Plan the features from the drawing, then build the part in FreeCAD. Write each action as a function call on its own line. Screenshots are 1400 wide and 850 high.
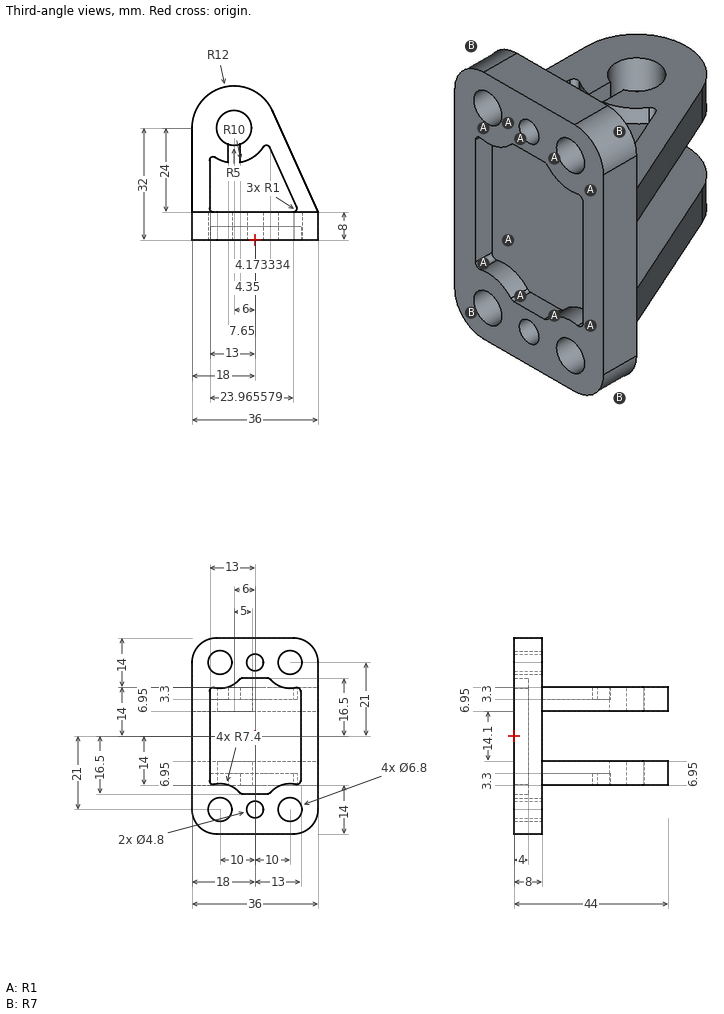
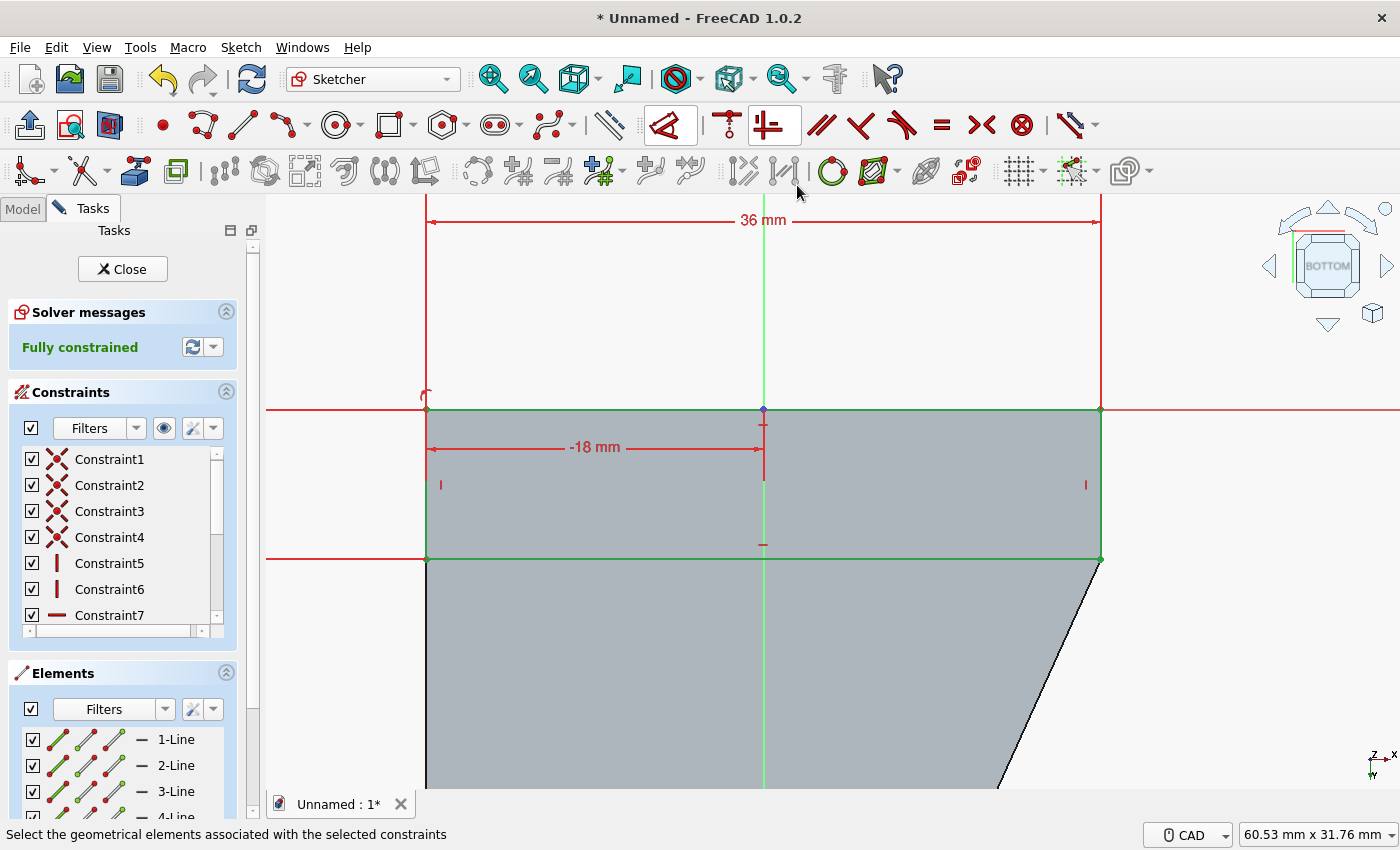
click(123, 269)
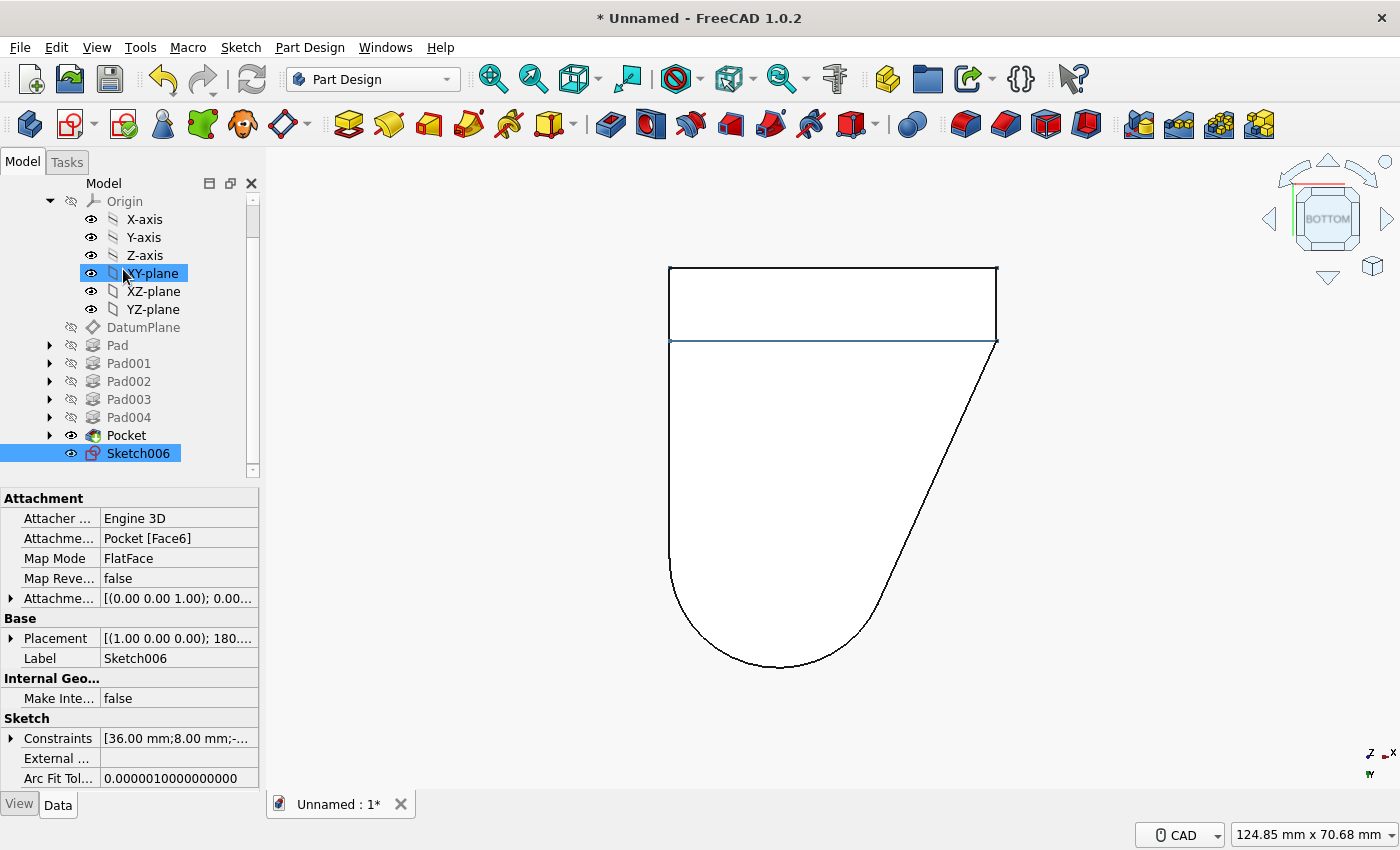
click(350, 124)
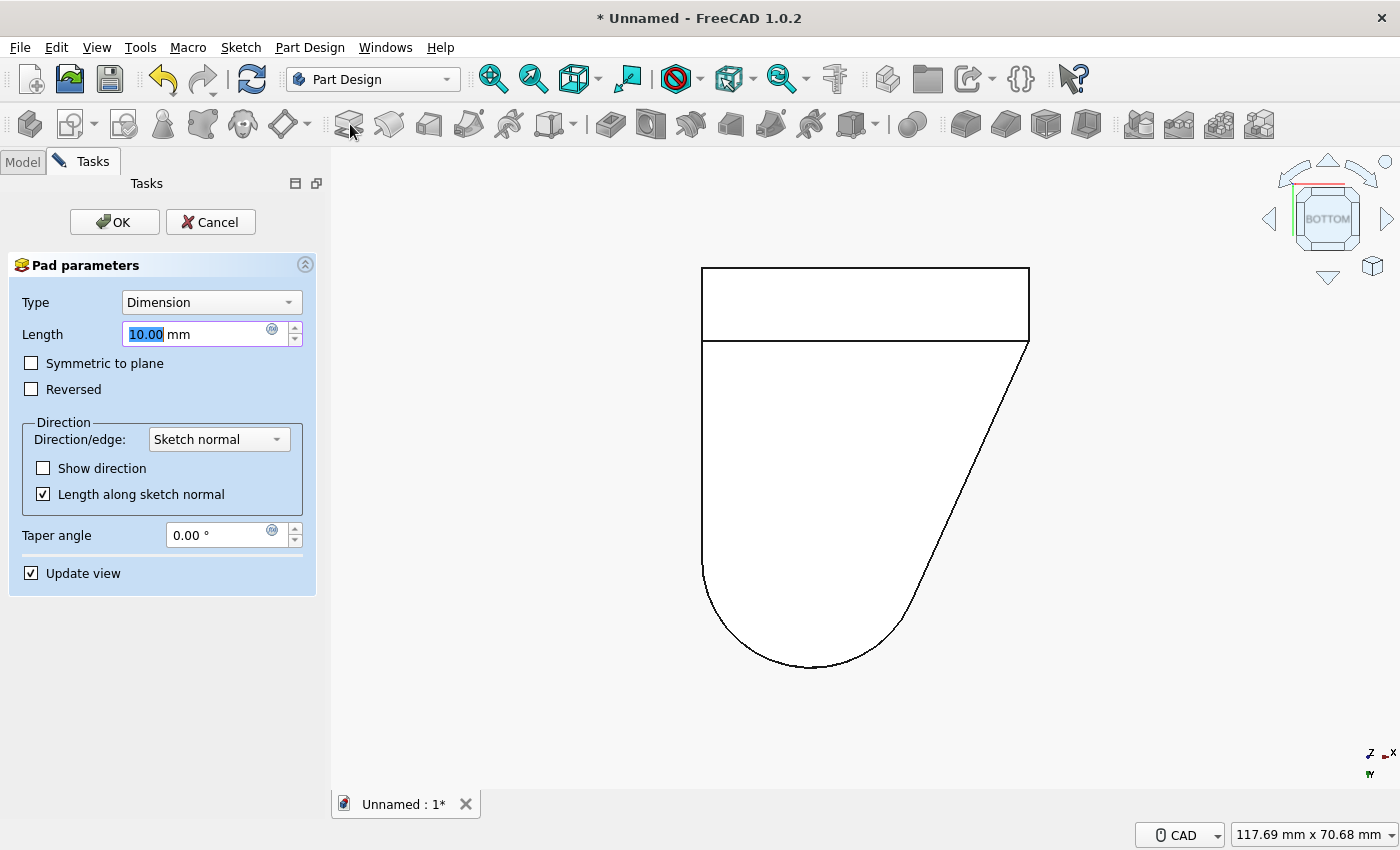
text(14)
key(Tab)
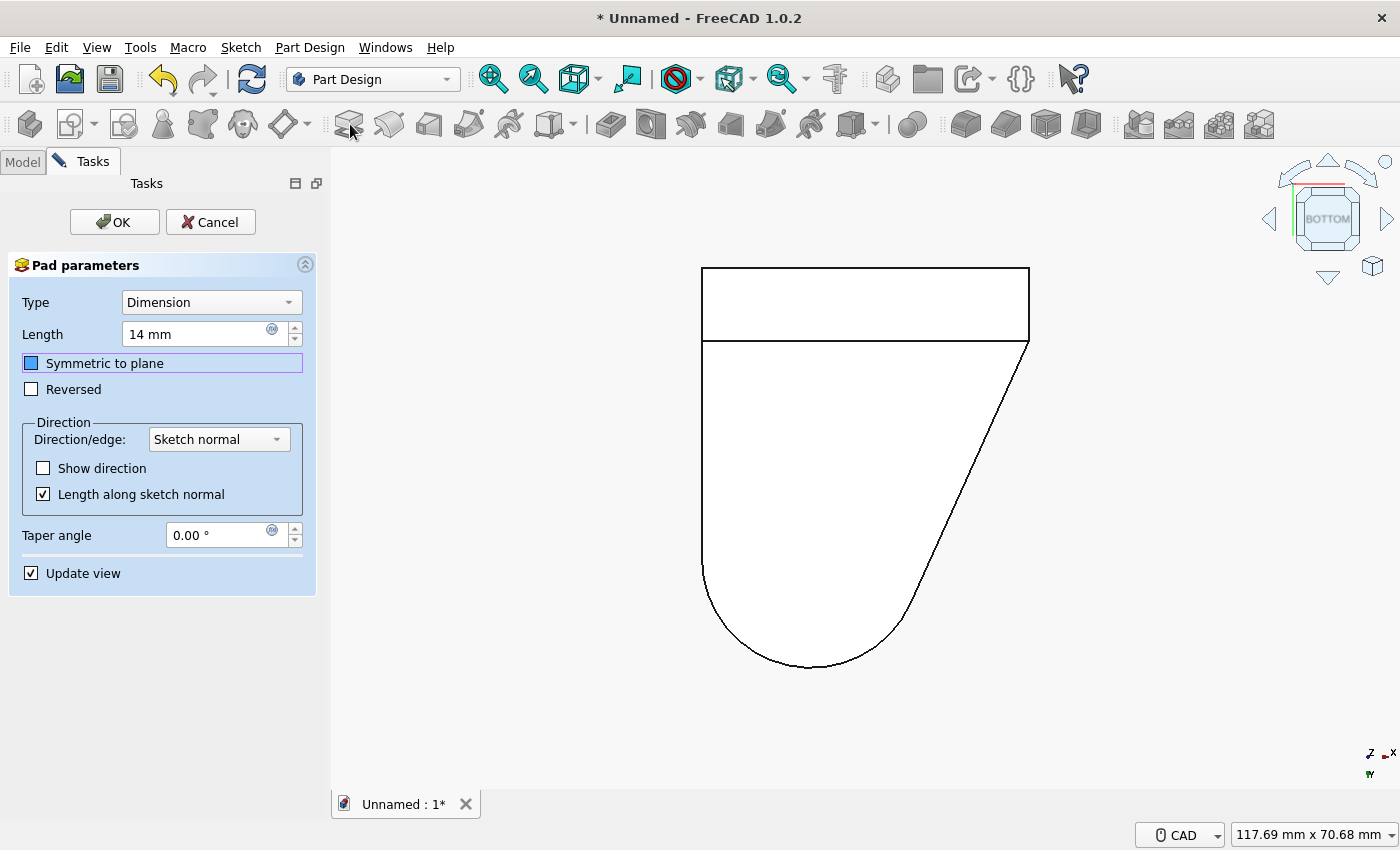
click(115, 222)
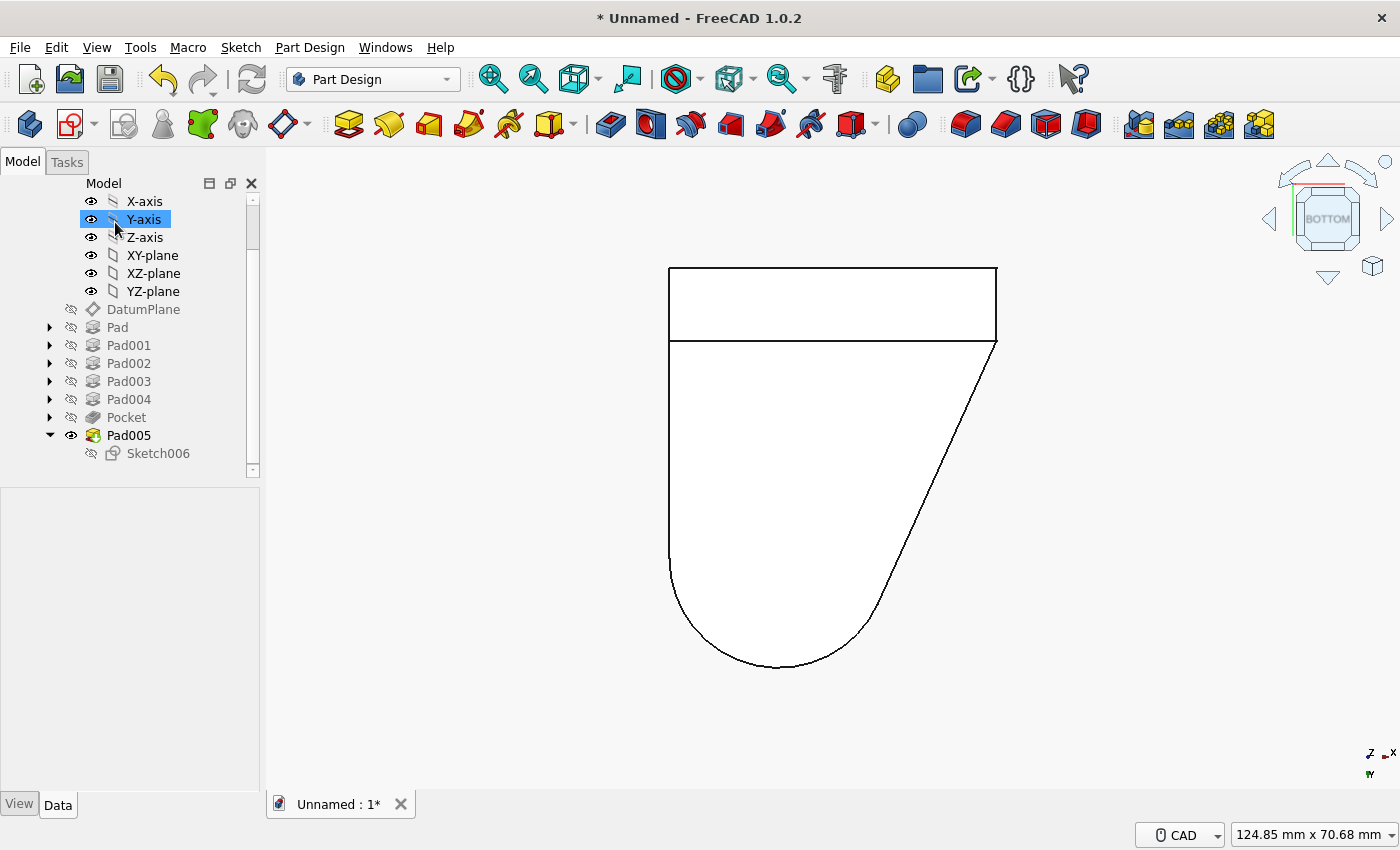
scroll(160, 323, down, 3)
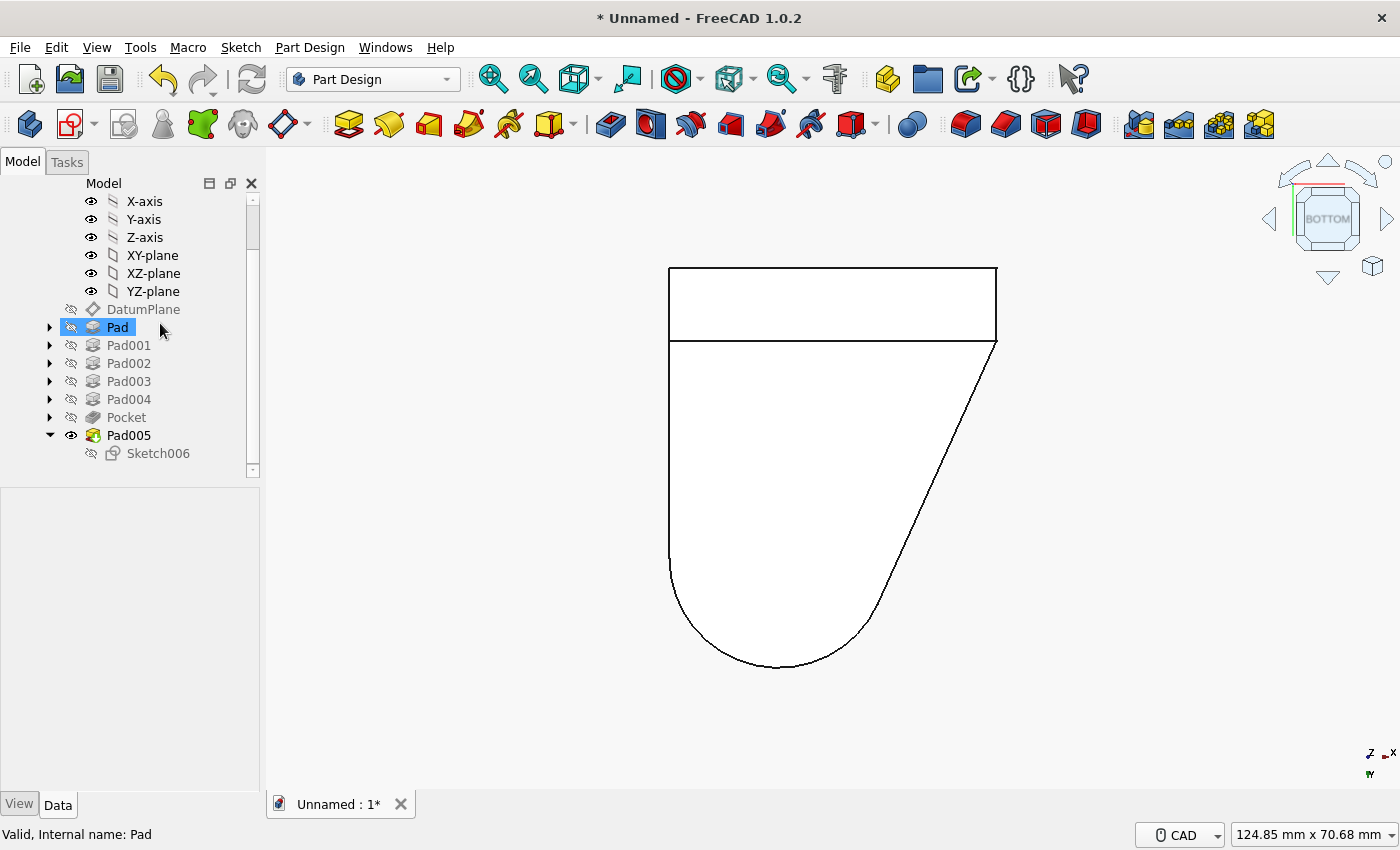
scroll(160, 323, up, 15)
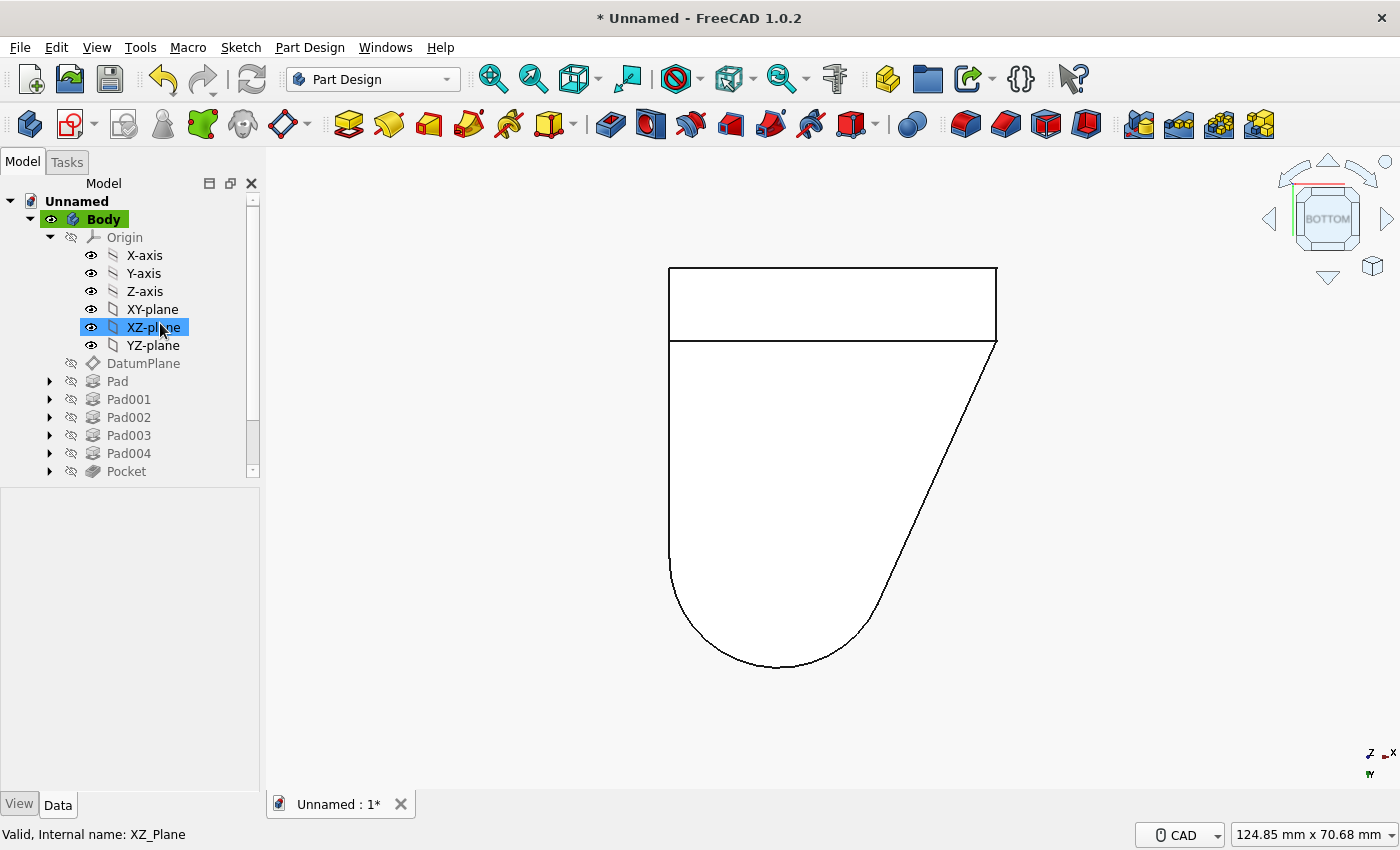
click(136, 309)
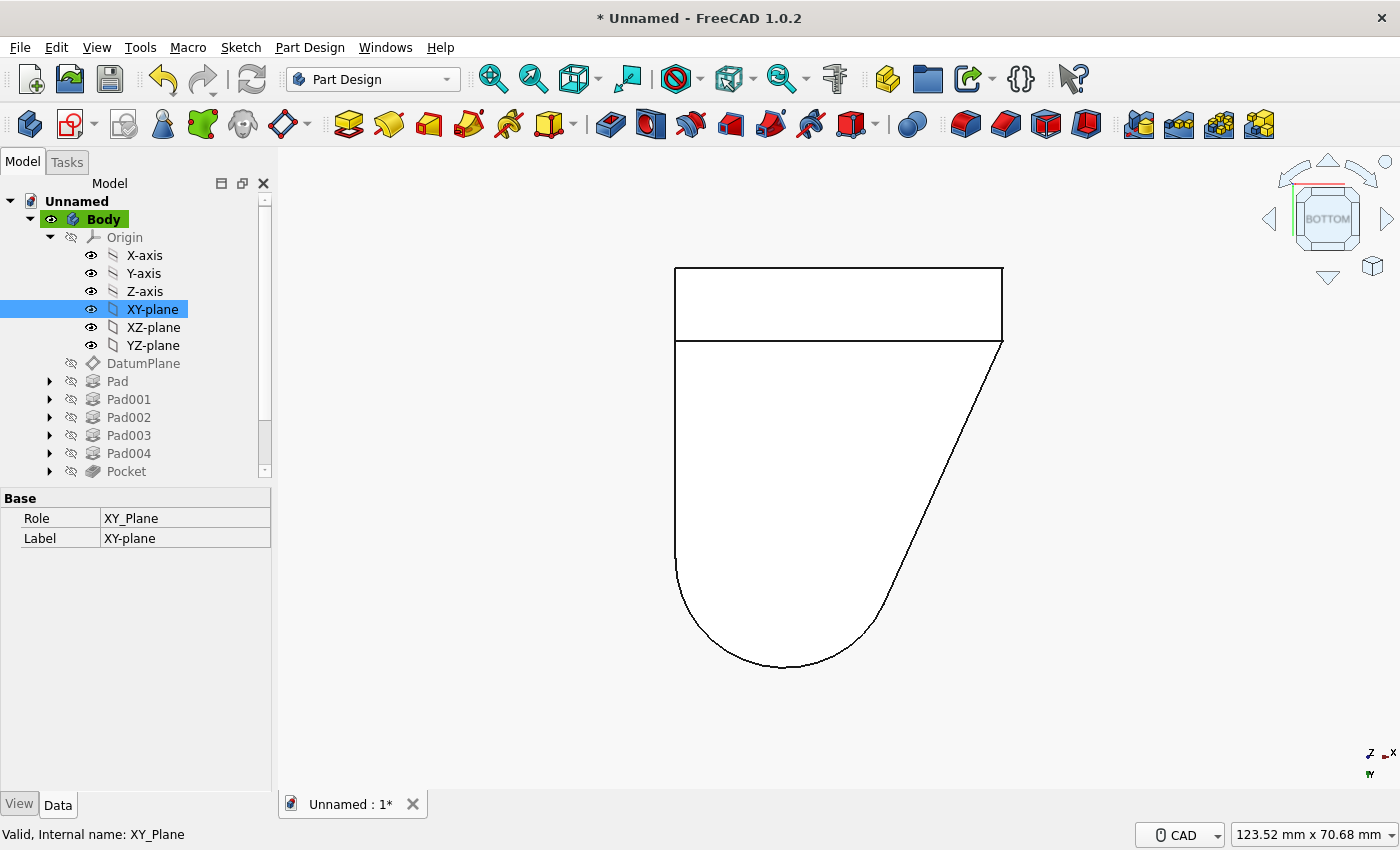
click(284, 124)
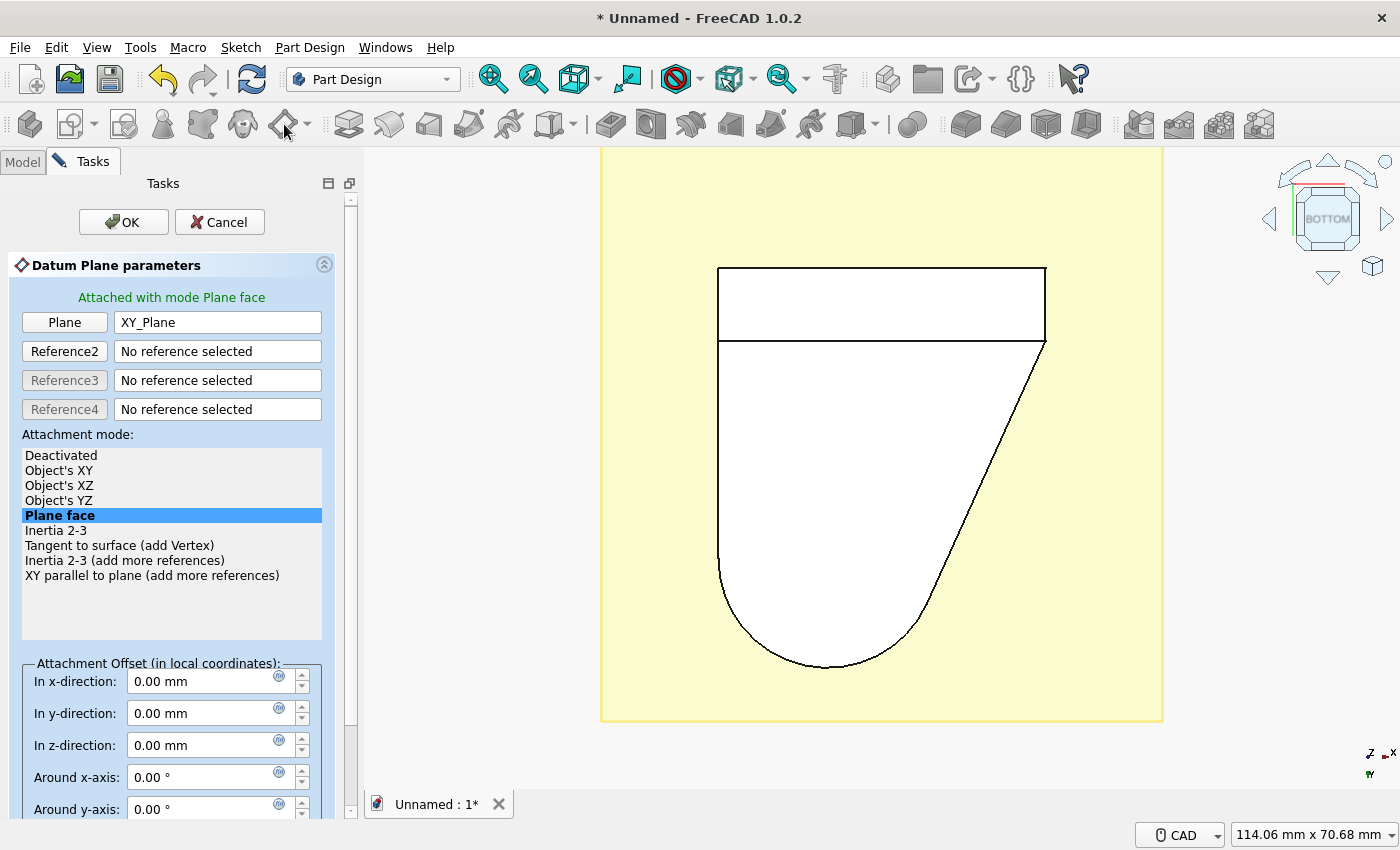
triple_click(210, 745)